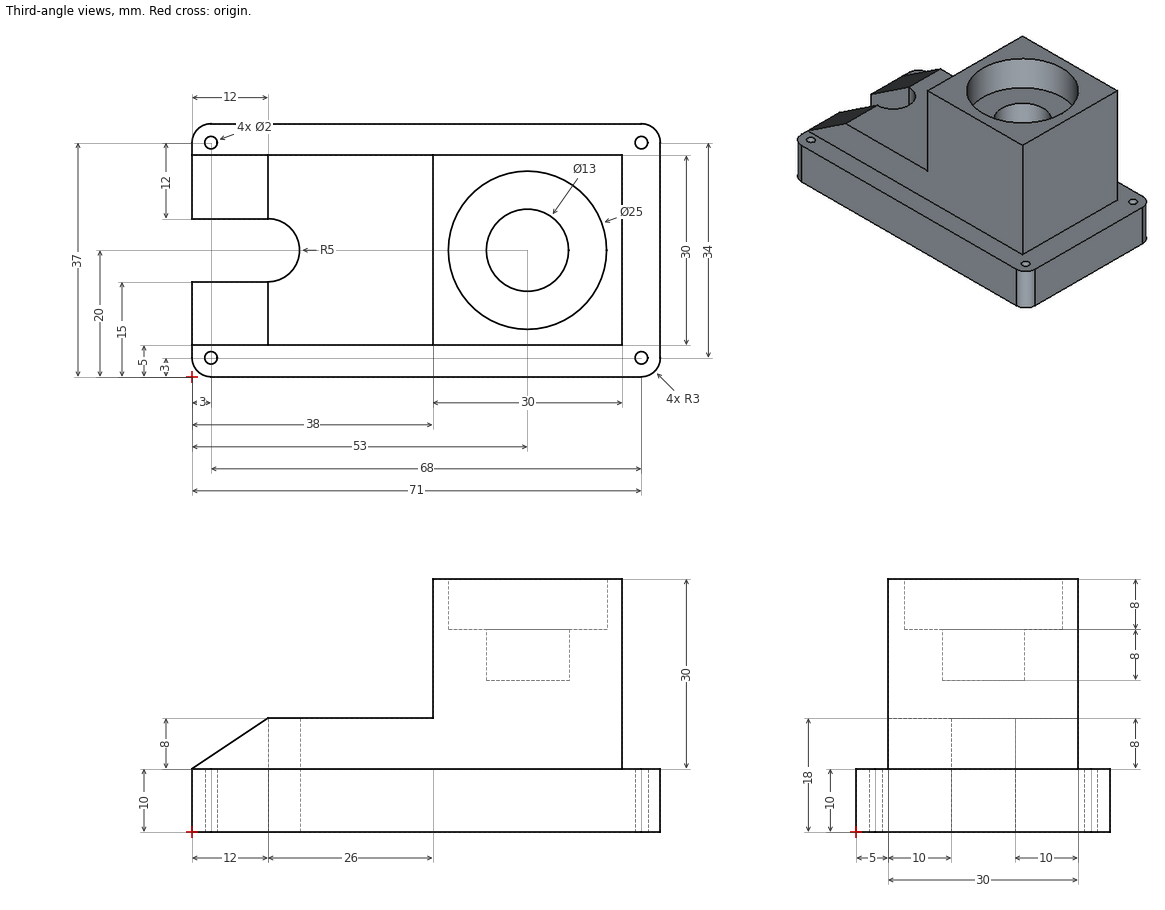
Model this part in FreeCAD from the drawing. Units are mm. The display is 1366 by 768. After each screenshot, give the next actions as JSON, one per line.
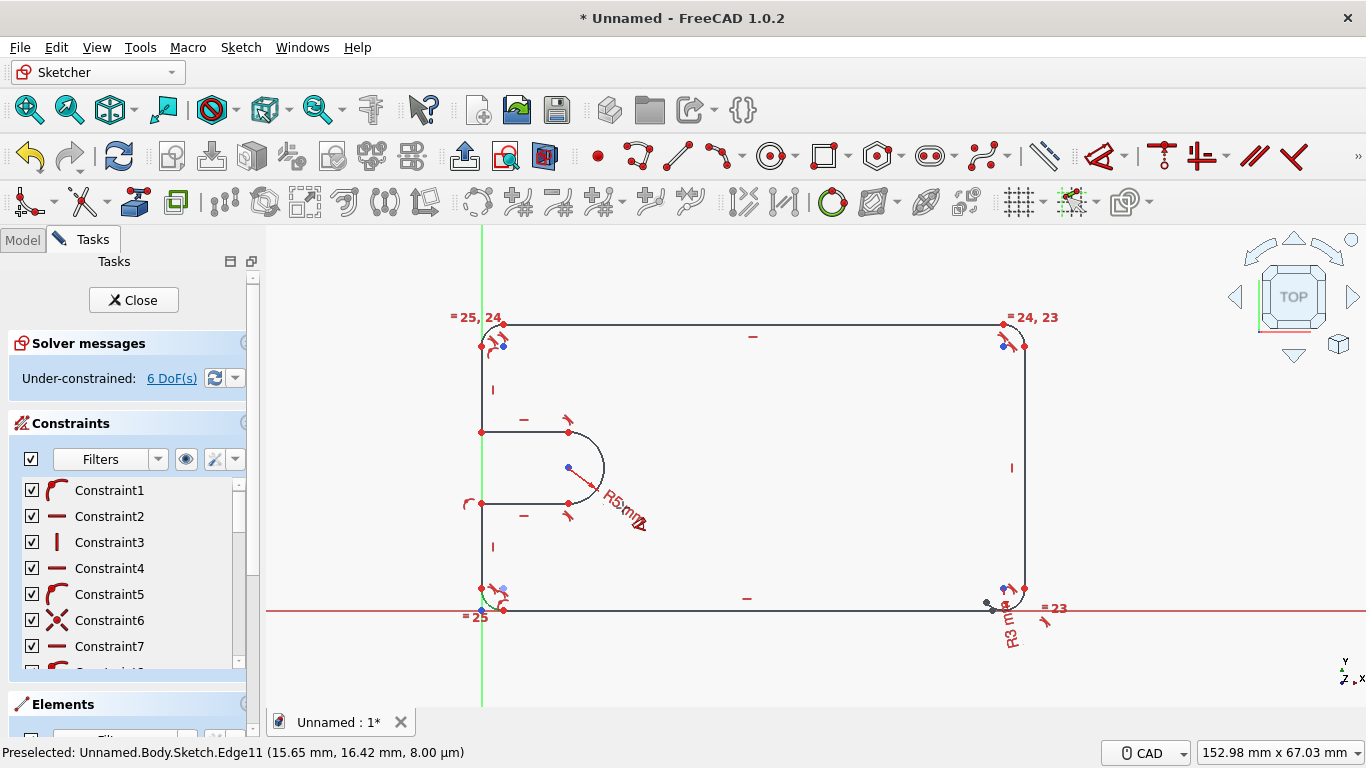
{"action": "left_click", "coordinate": [650, 611]}
{"action": "left_click", "coordinate": [748, 645]}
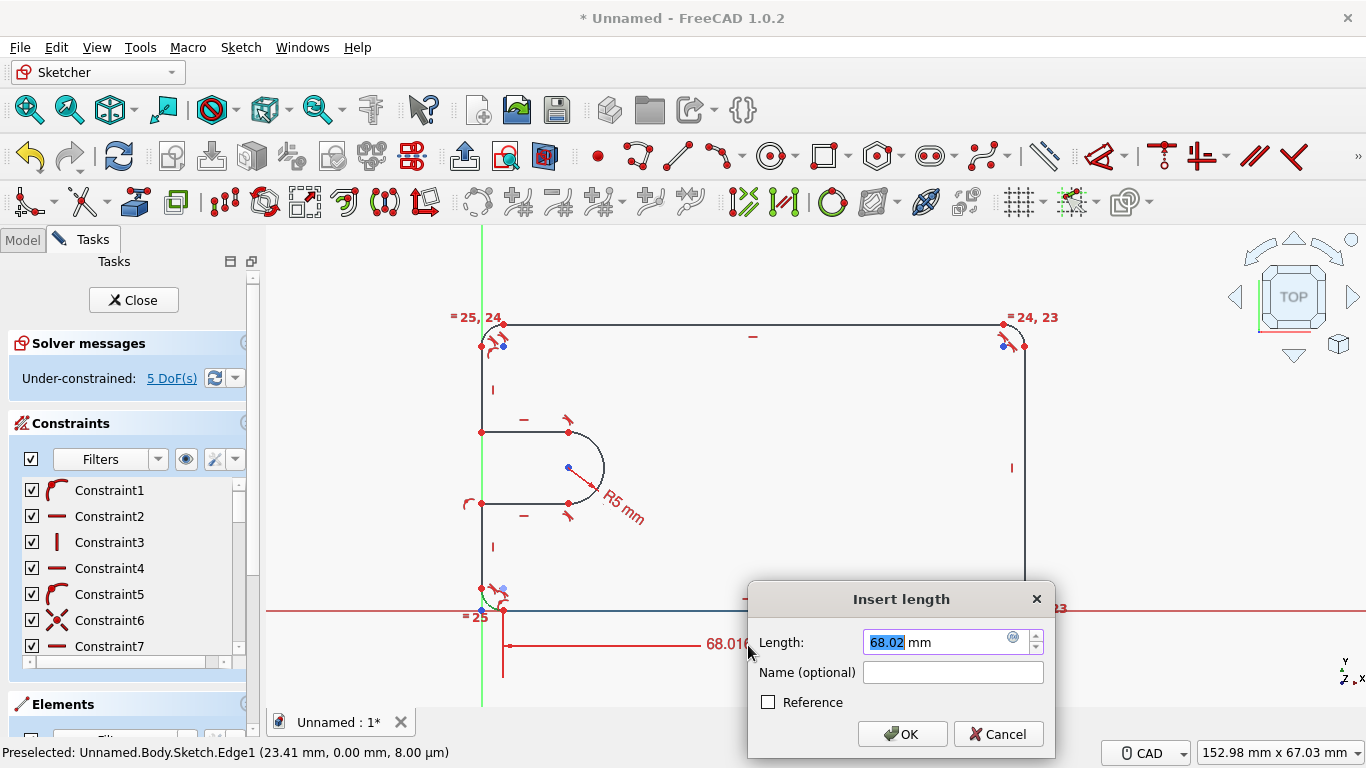
{"action": "type", "text": "68"}
{"action": "key", "text": "Return"}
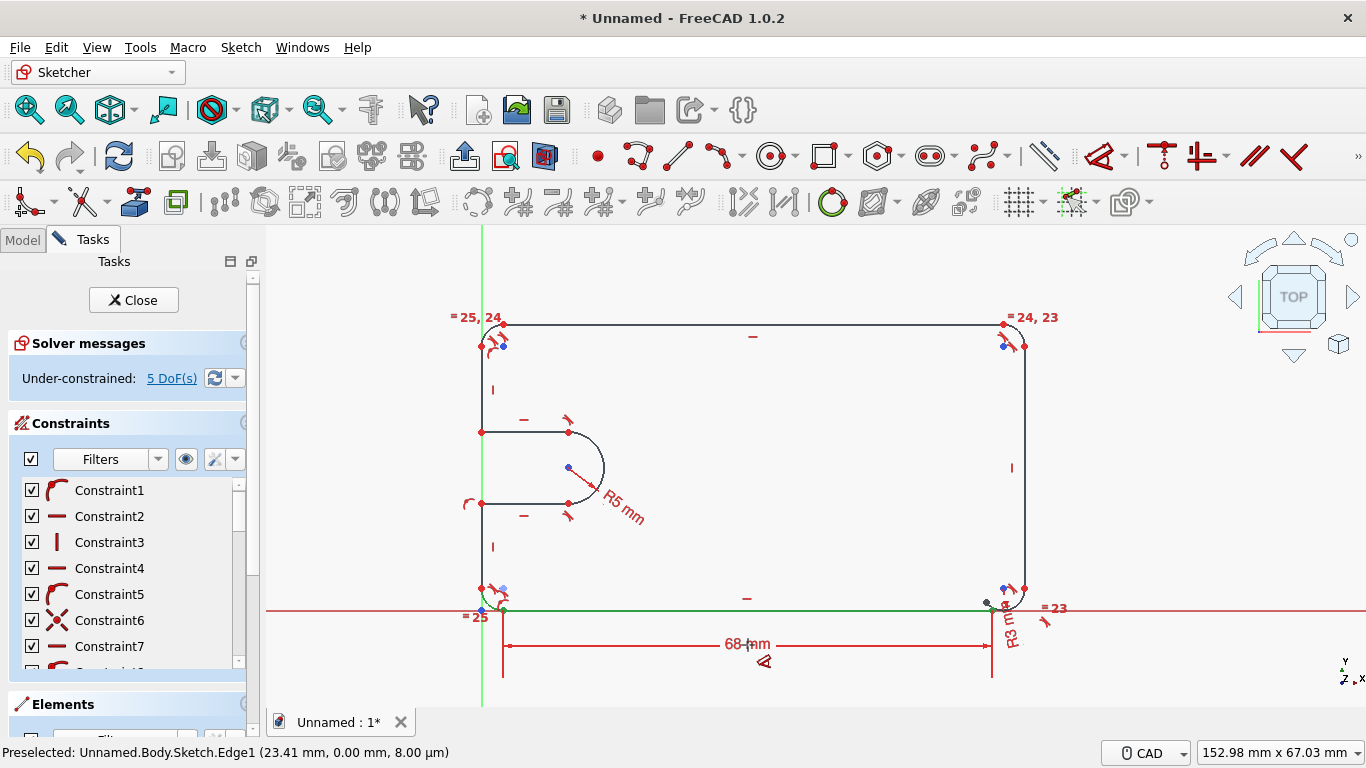
{"action": "left_click", "coordinate": [1025, 516]}
{"action": "left_click", "coordinate": [1059, 468]}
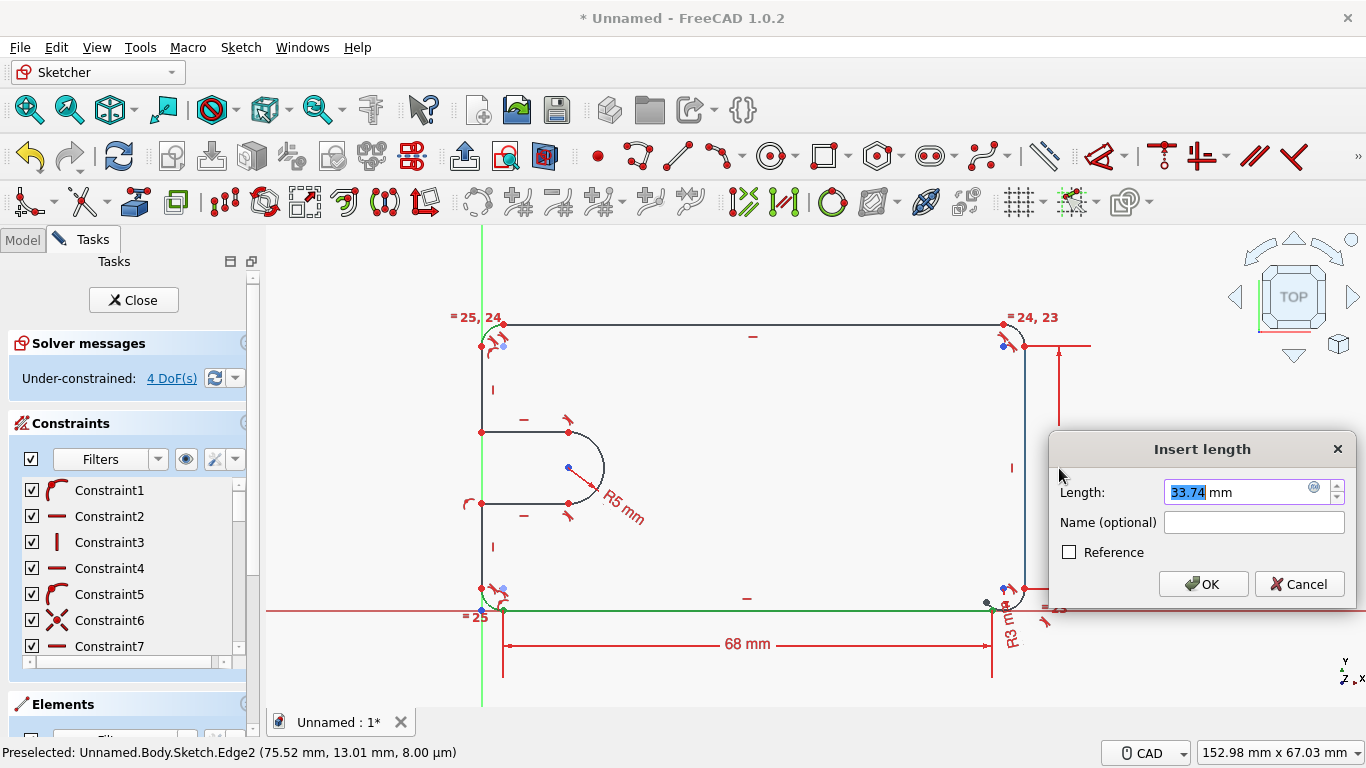
{"action": "type", "text": "34"}
{"action": "key", "text": "Return"}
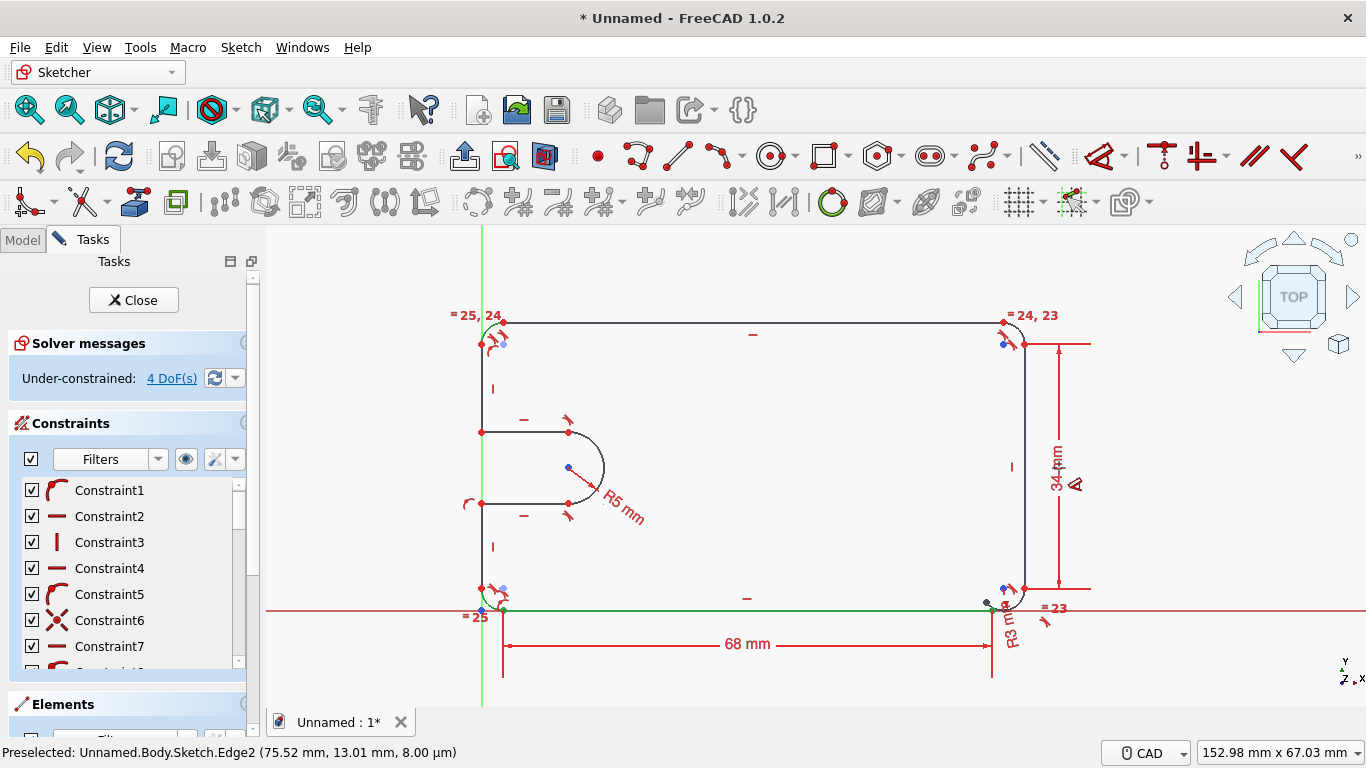
{"action": "left_click", "coordinate": [853, 323]}
{"action": "left_click", "coordinate": [753, 289]}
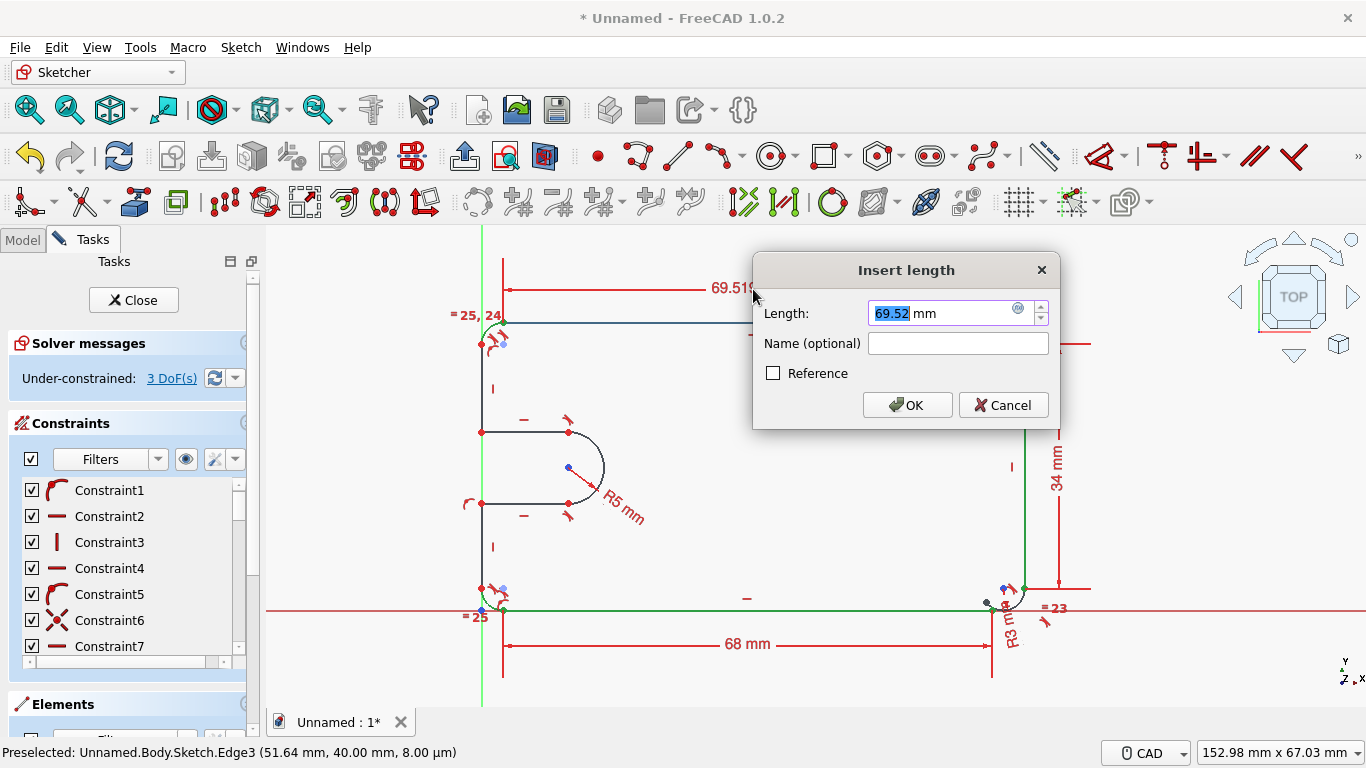
{"action": "type", "text": "68"}
{"action": "key", "text": "Return"}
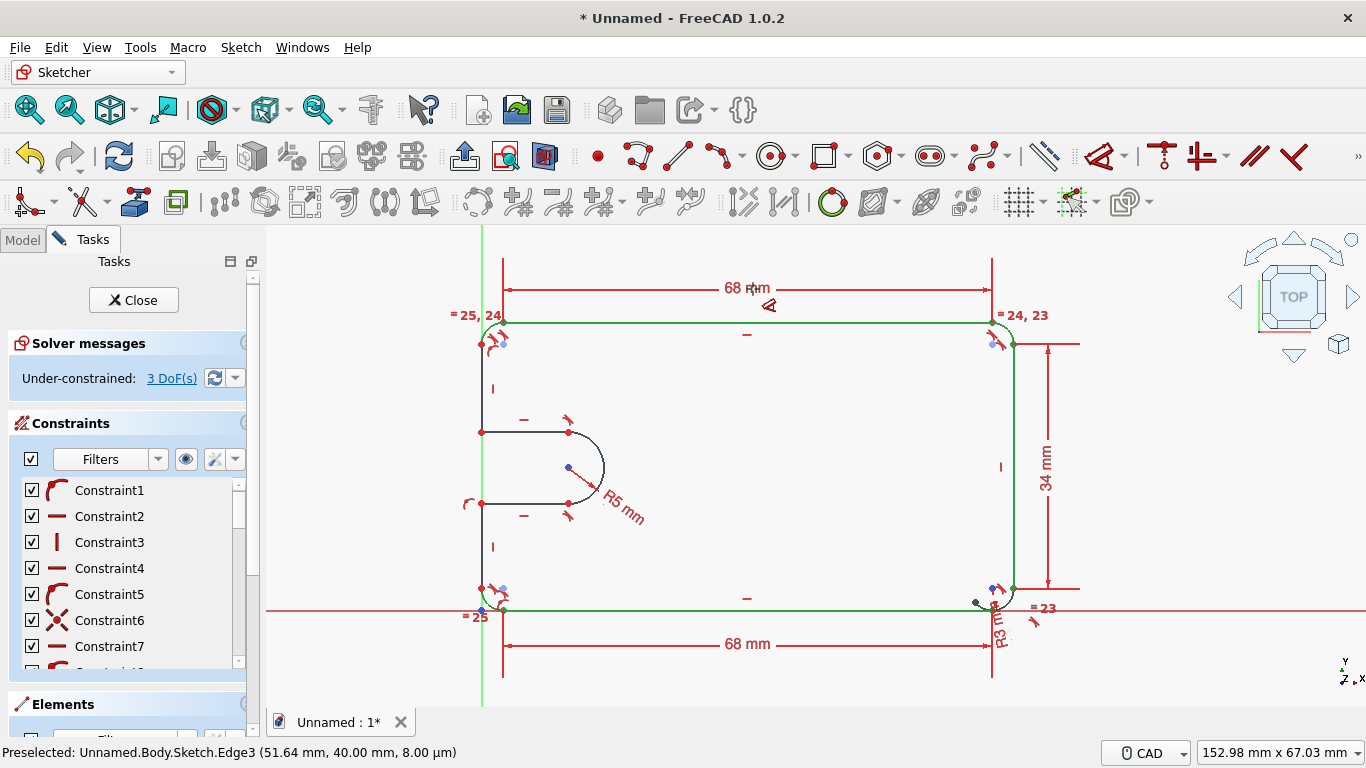
{"action": "left_click", "coordinate": [482, 371]}
{"action": "left_click", "coordinate": [448, 388]}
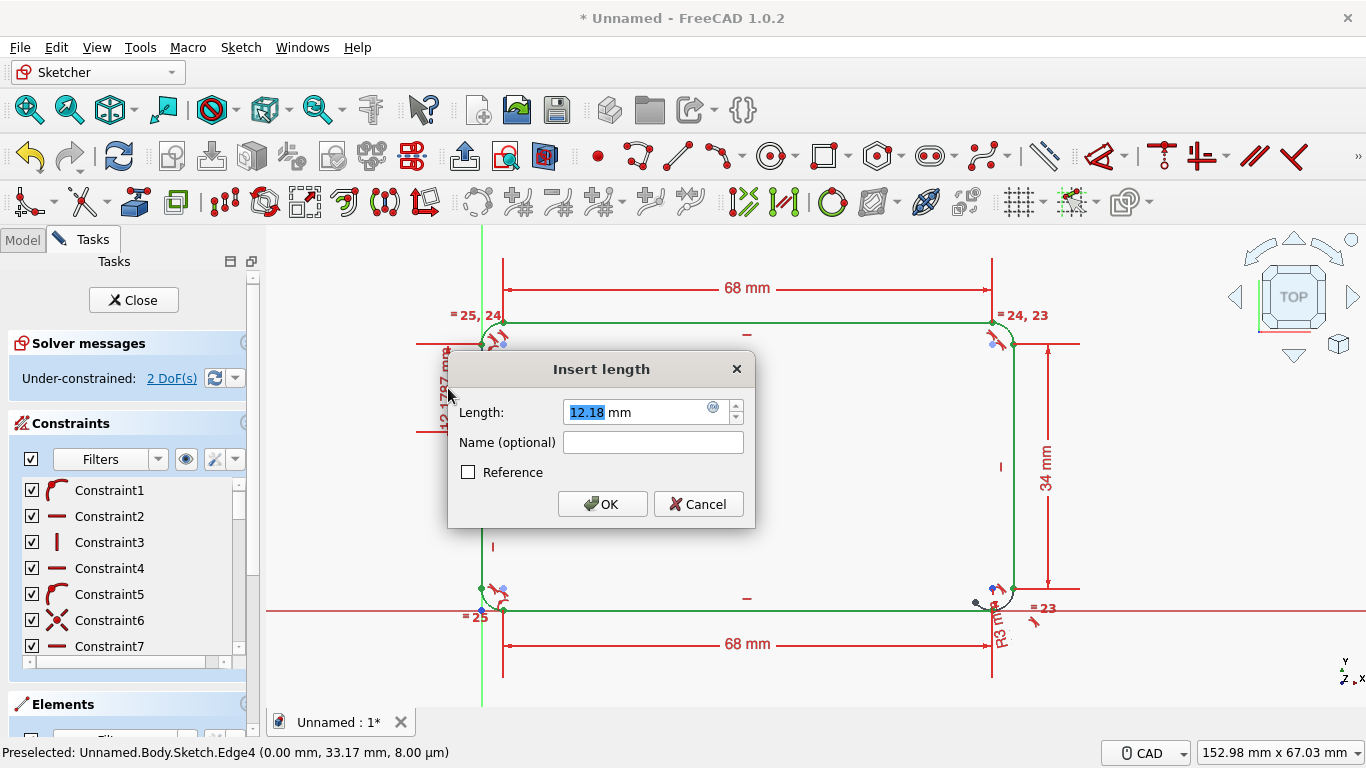
{"action": "type", "text": "12"}
{"action": "key", "text": "Return"}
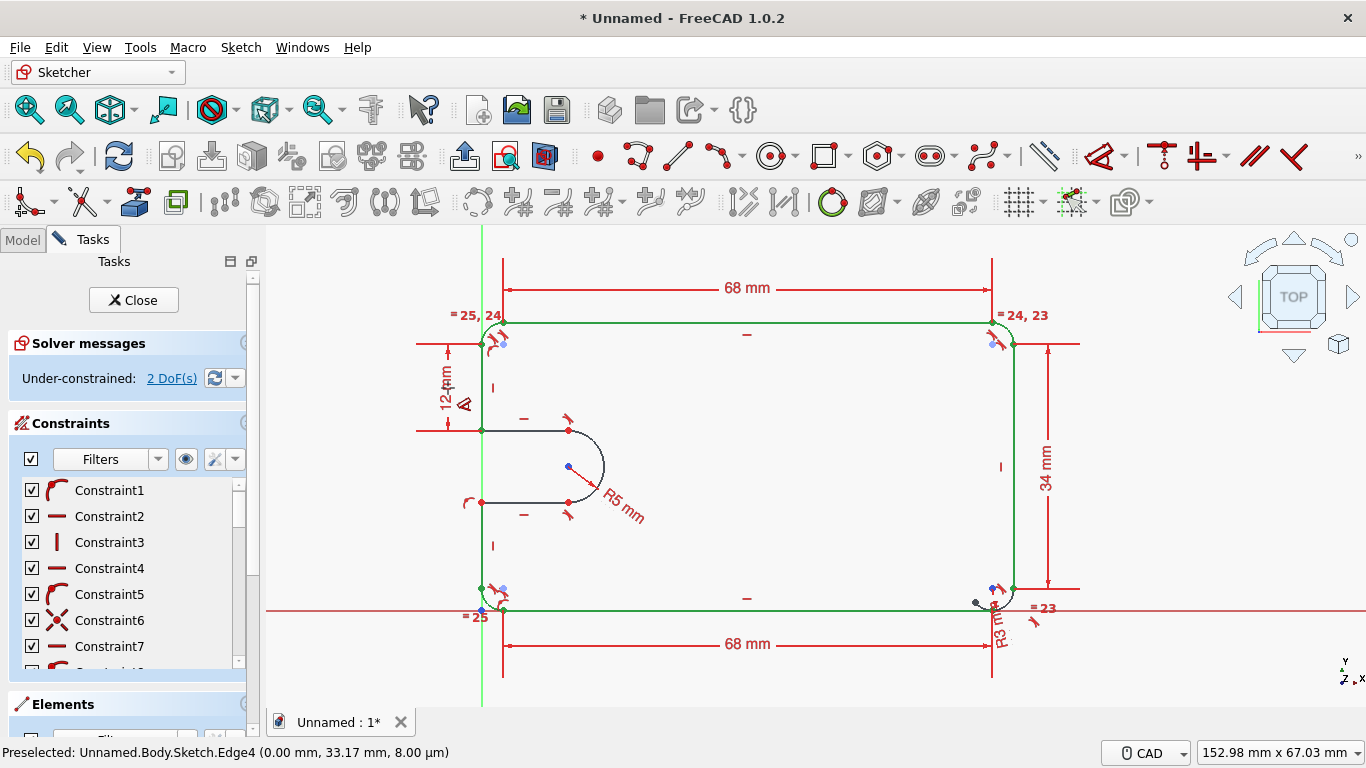
{"action": "left_click", "coordinate": [508, 431]}
{"action": "left_click", "coordinate": [525, 397]}